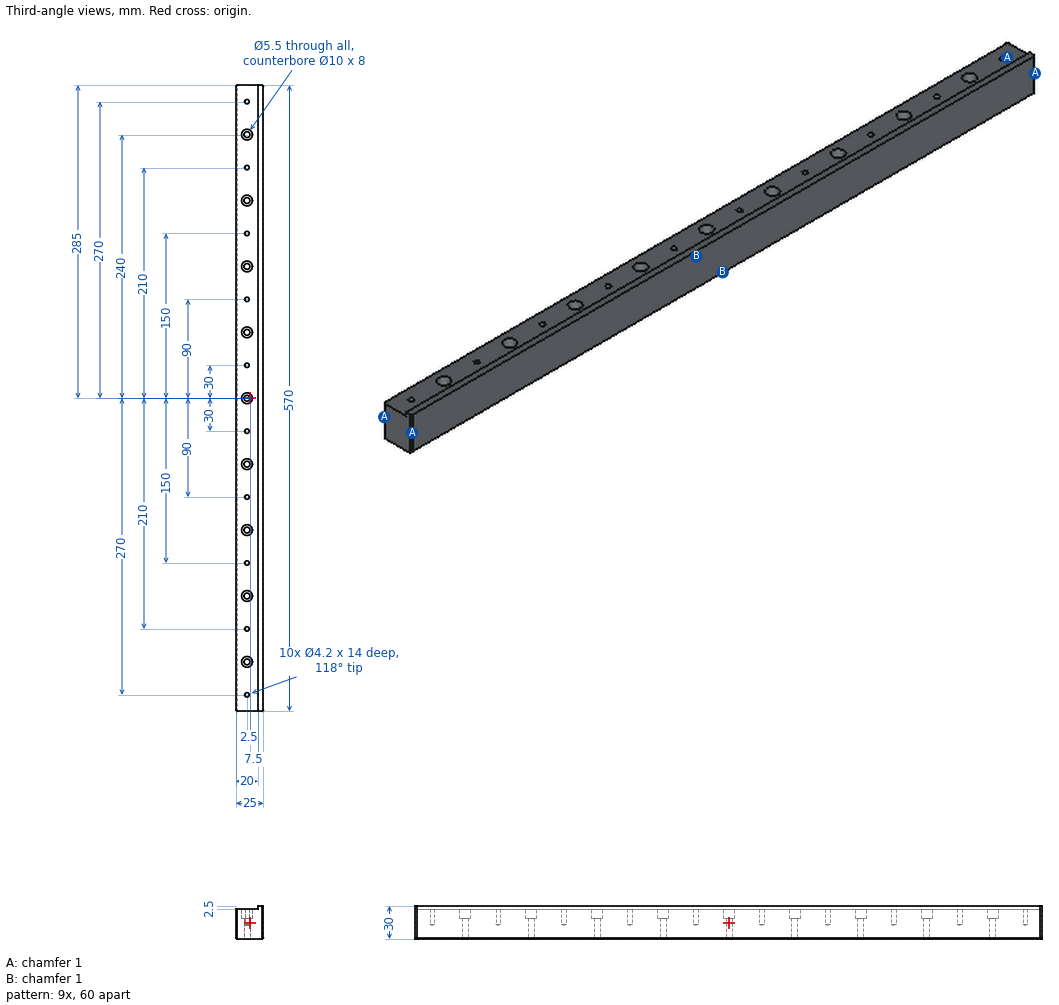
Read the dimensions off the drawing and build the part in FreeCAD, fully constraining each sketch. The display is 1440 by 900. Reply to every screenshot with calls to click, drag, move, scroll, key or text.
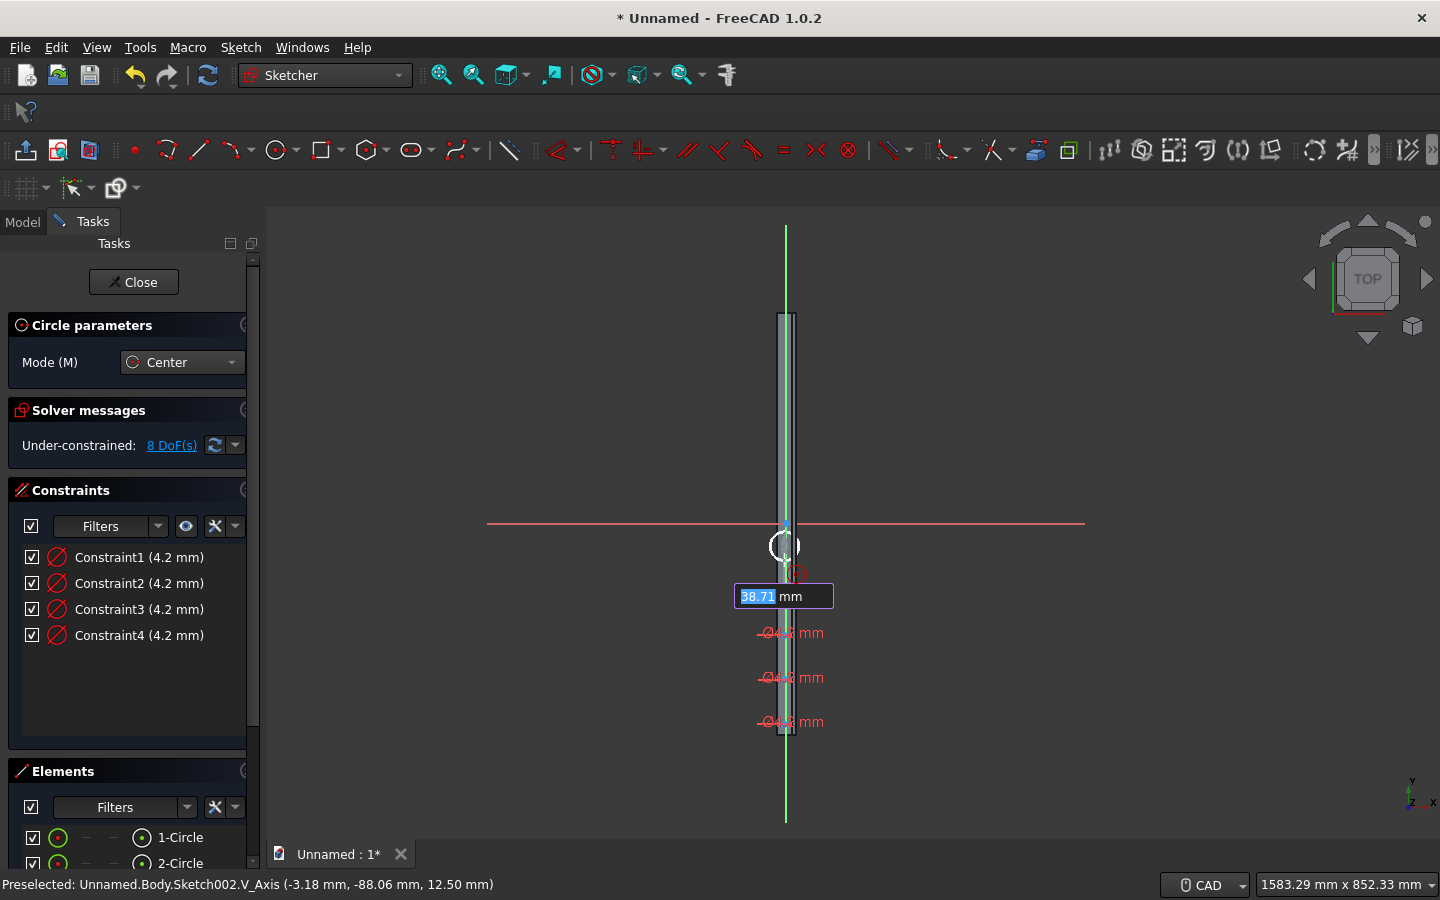
scroll(783, 545, up, 9)
move(783, 543)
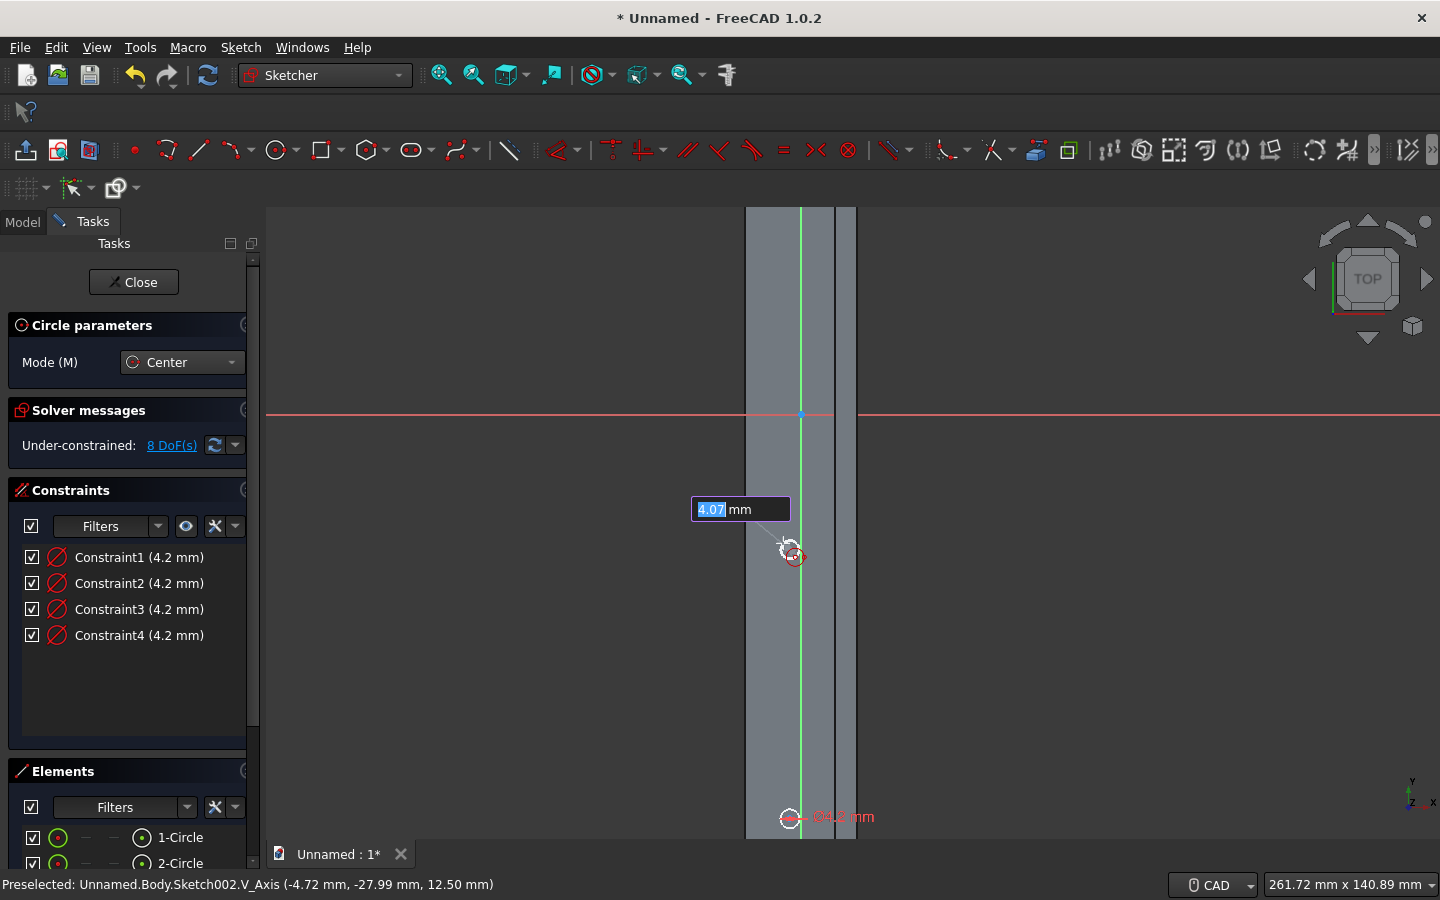
text(4.2)
key(Return)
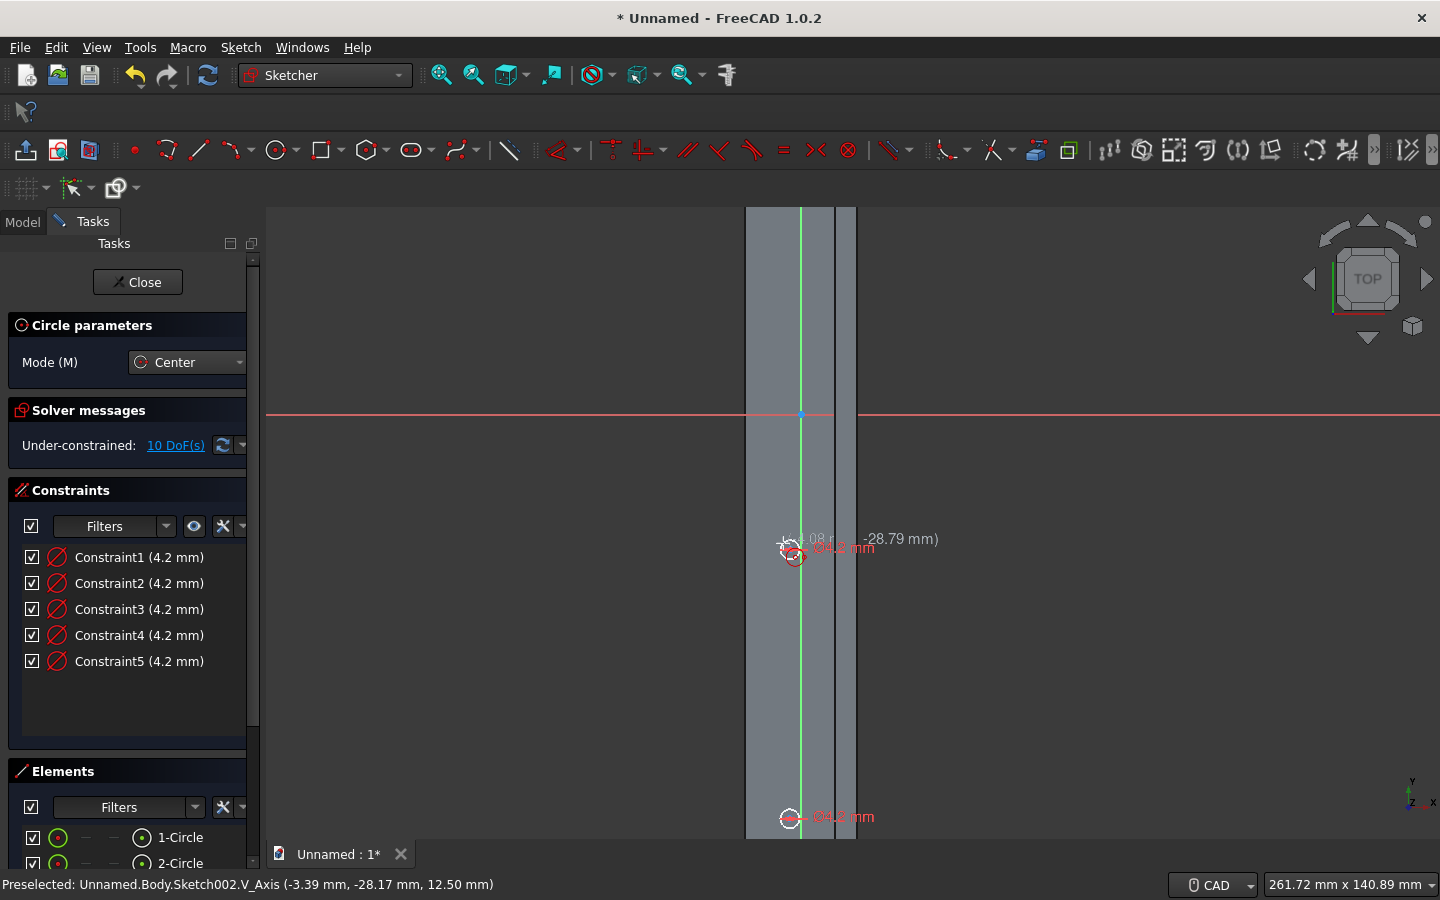
scroll(790, 280, up, 5)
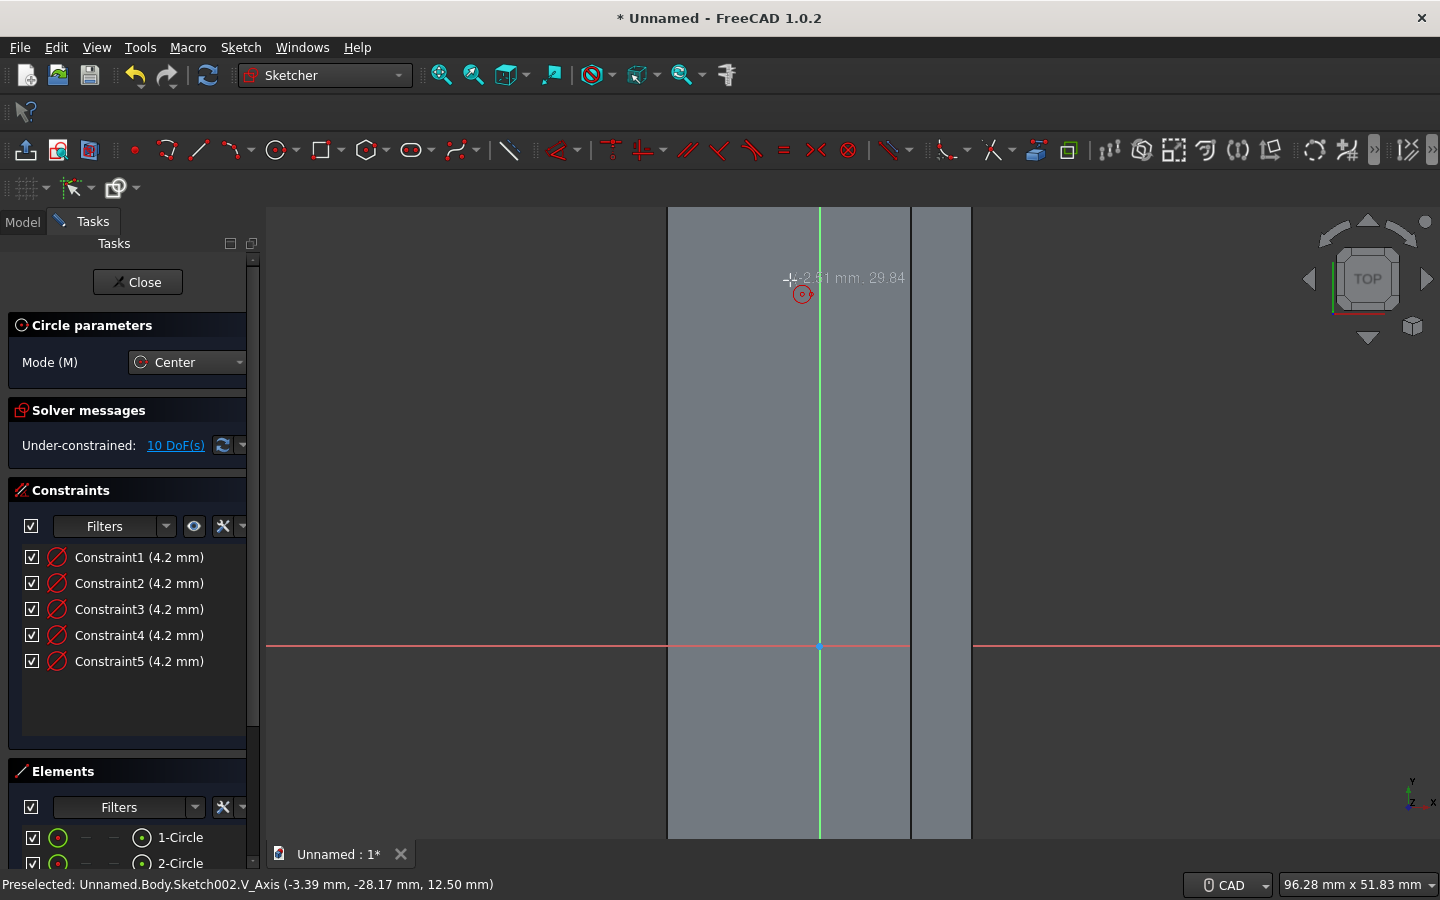
click(789, 281)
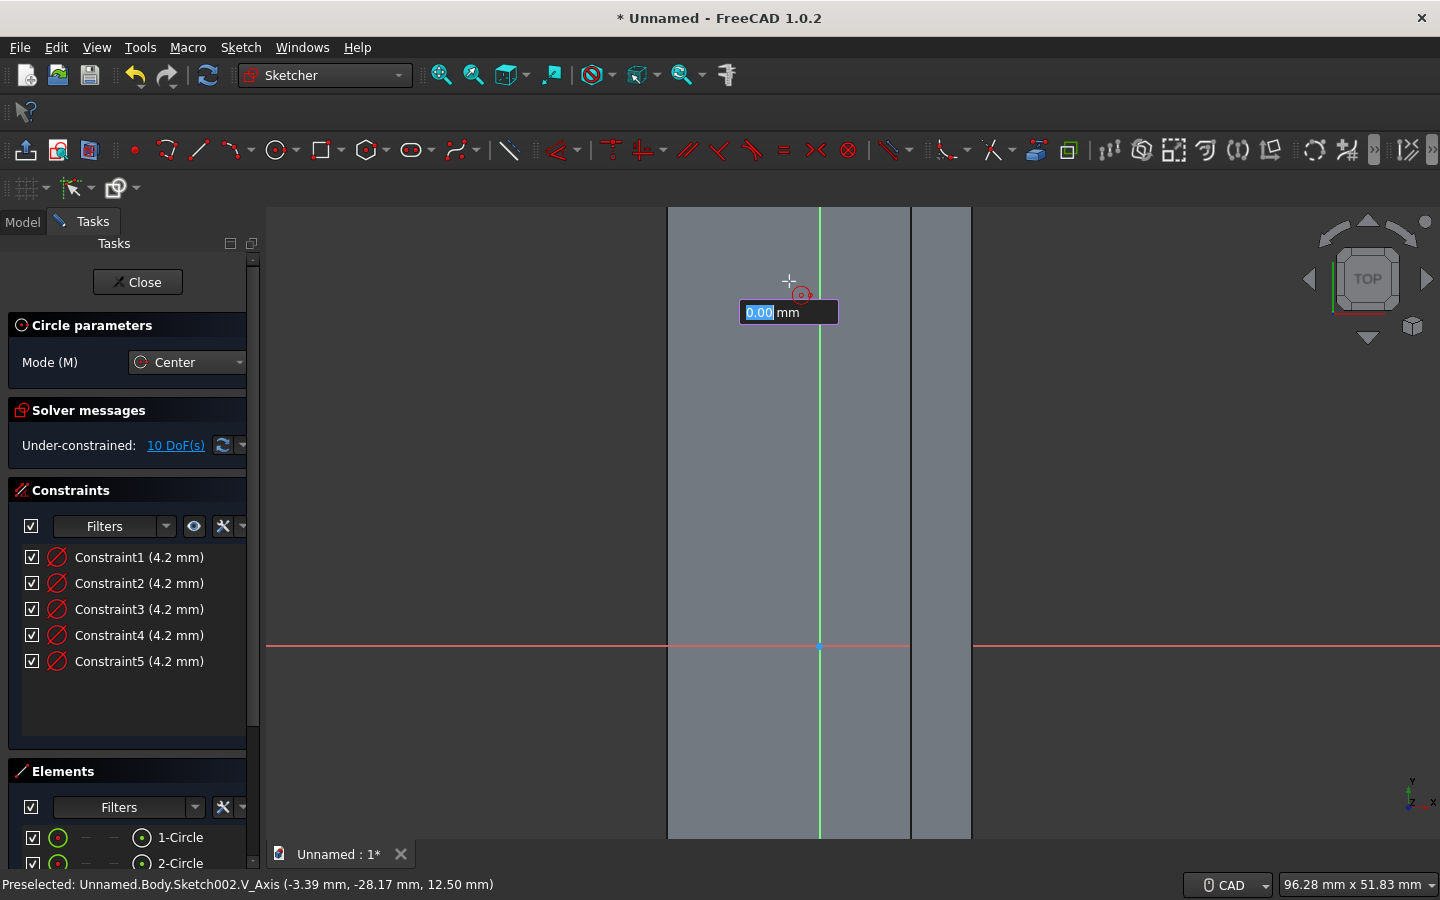
scroll(784, 515, down, 14)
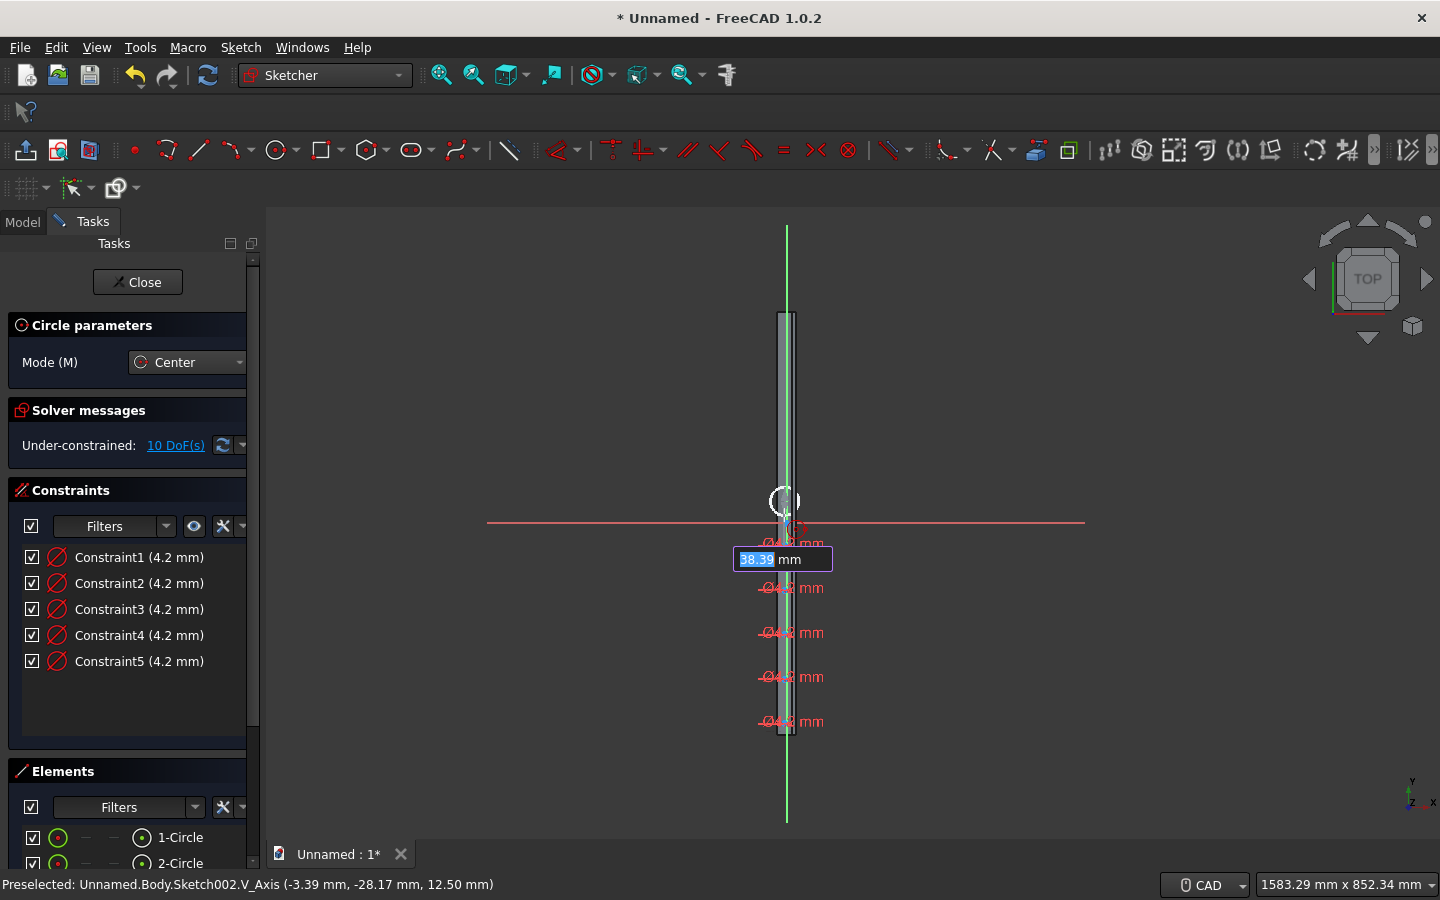
scroll(784, 500, up, 9)
move(780, 498)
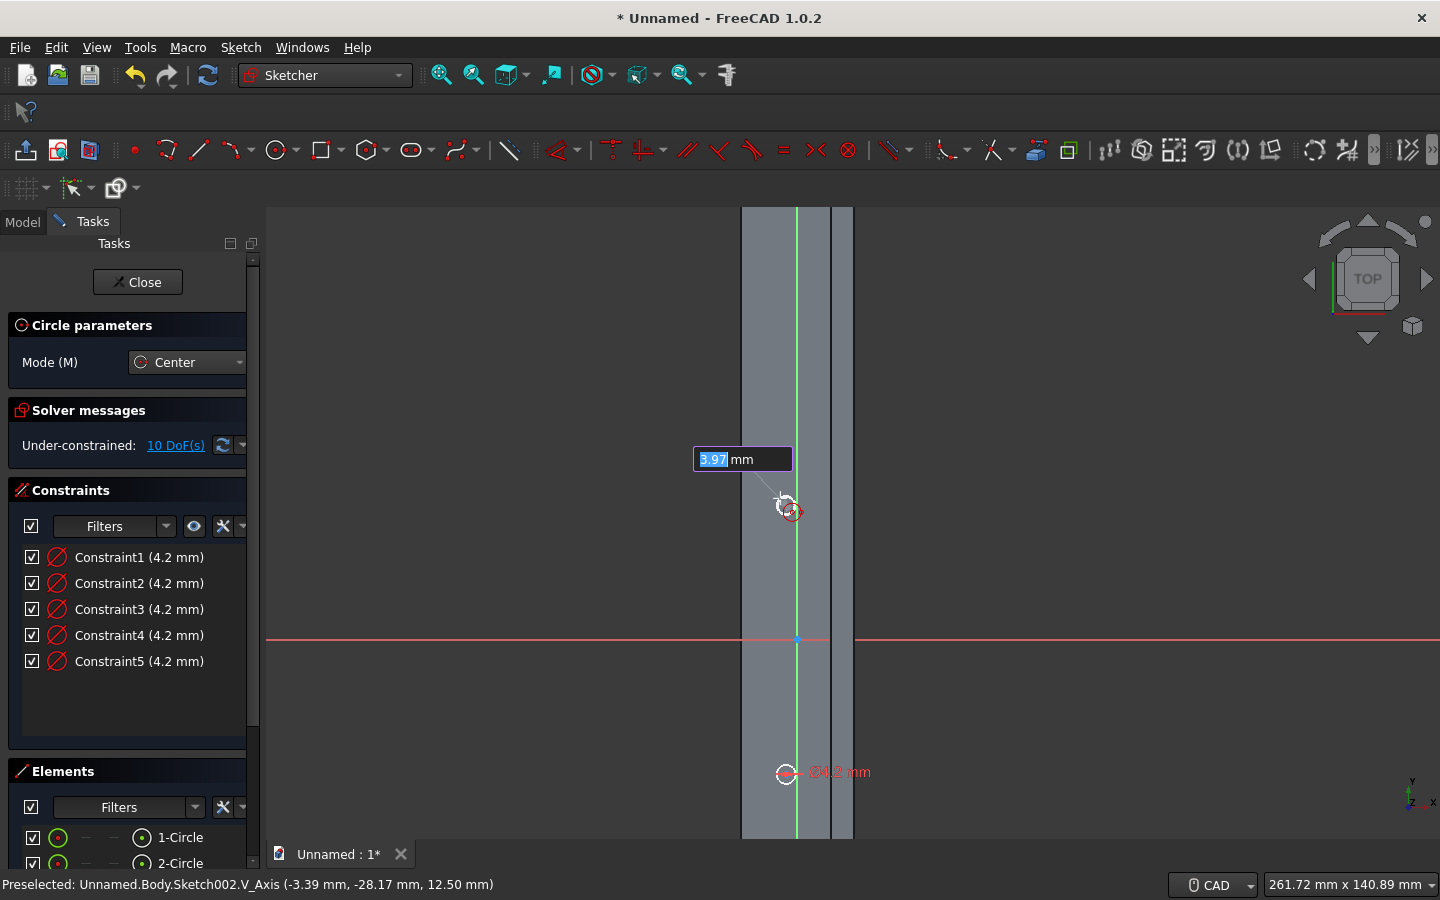
text(4.2)
key(Return)